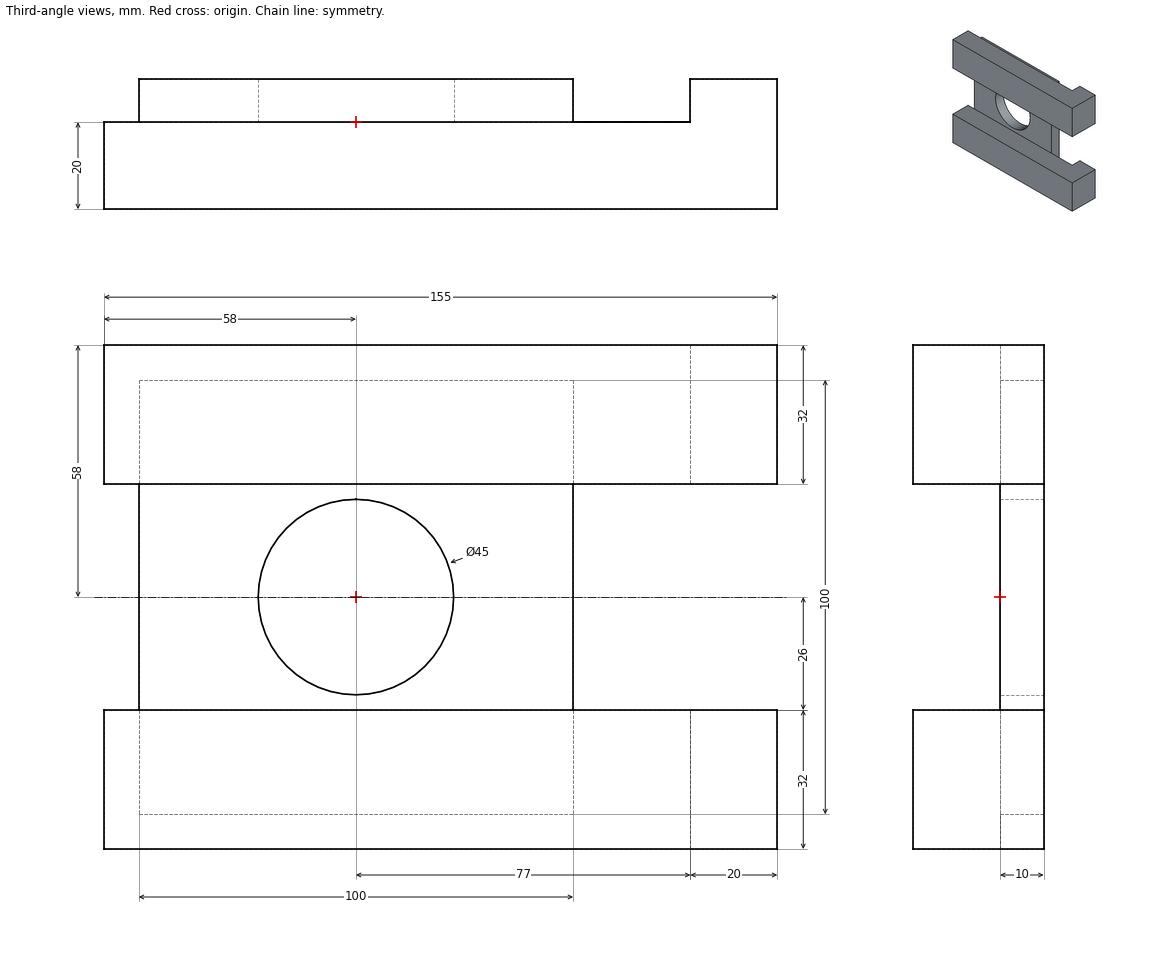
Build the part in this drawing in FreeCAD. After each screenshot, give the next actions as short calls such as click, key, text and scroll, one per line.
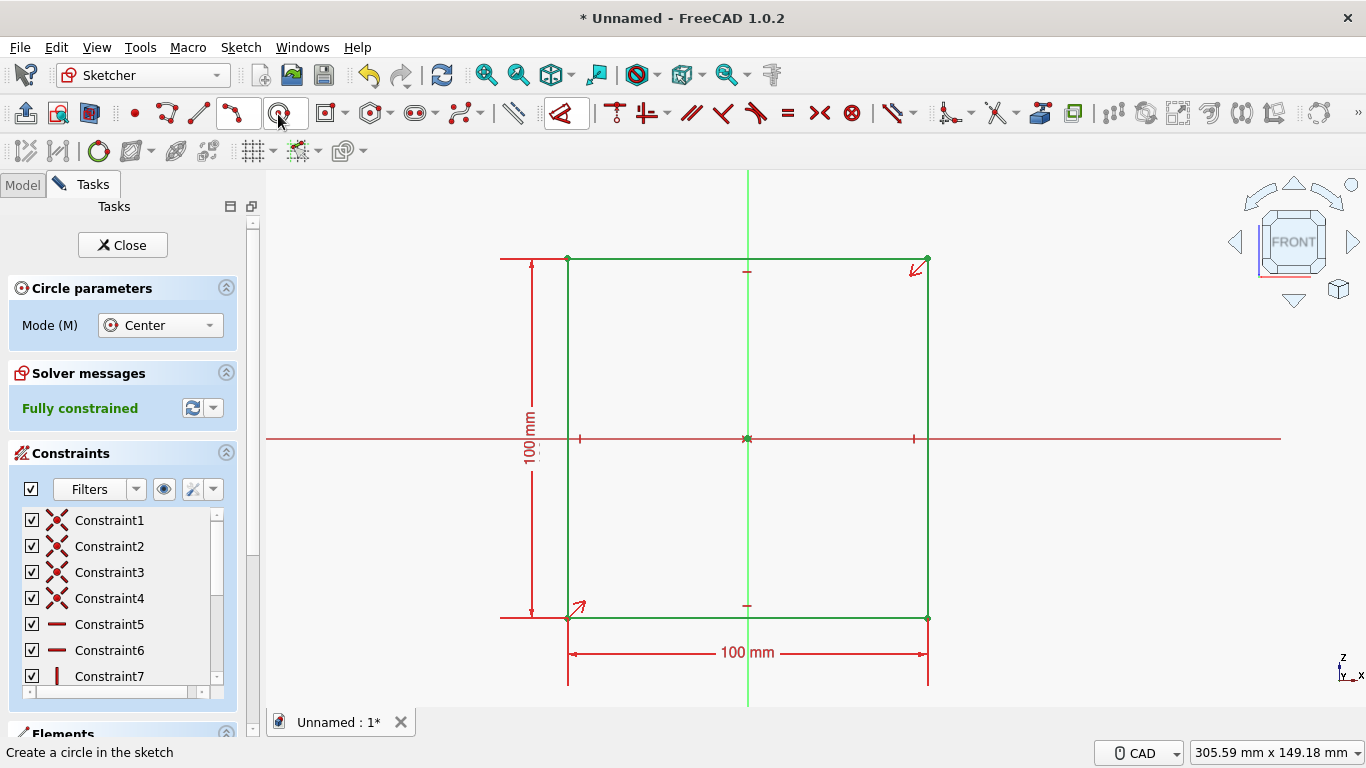
click(748, 438)
move(805, 381)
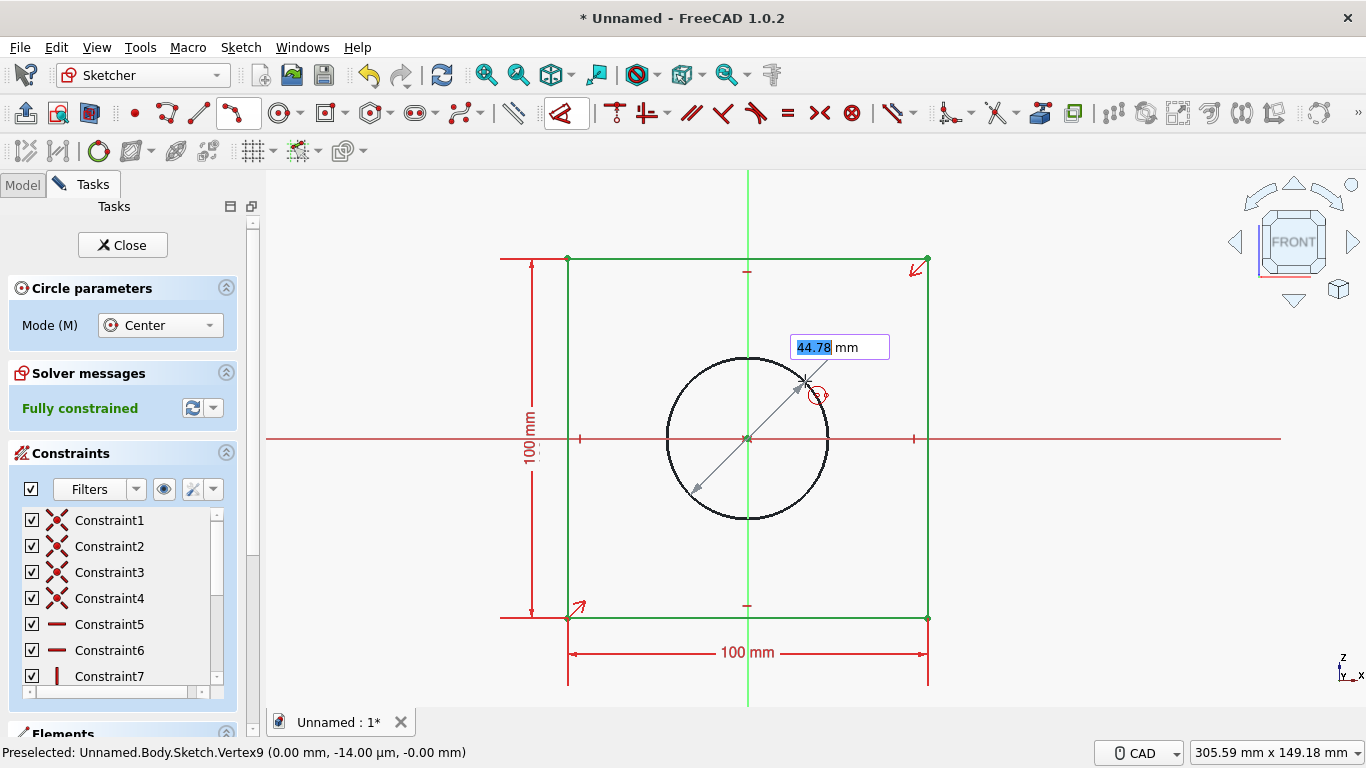
text(45)
key(Return)
key(Escape)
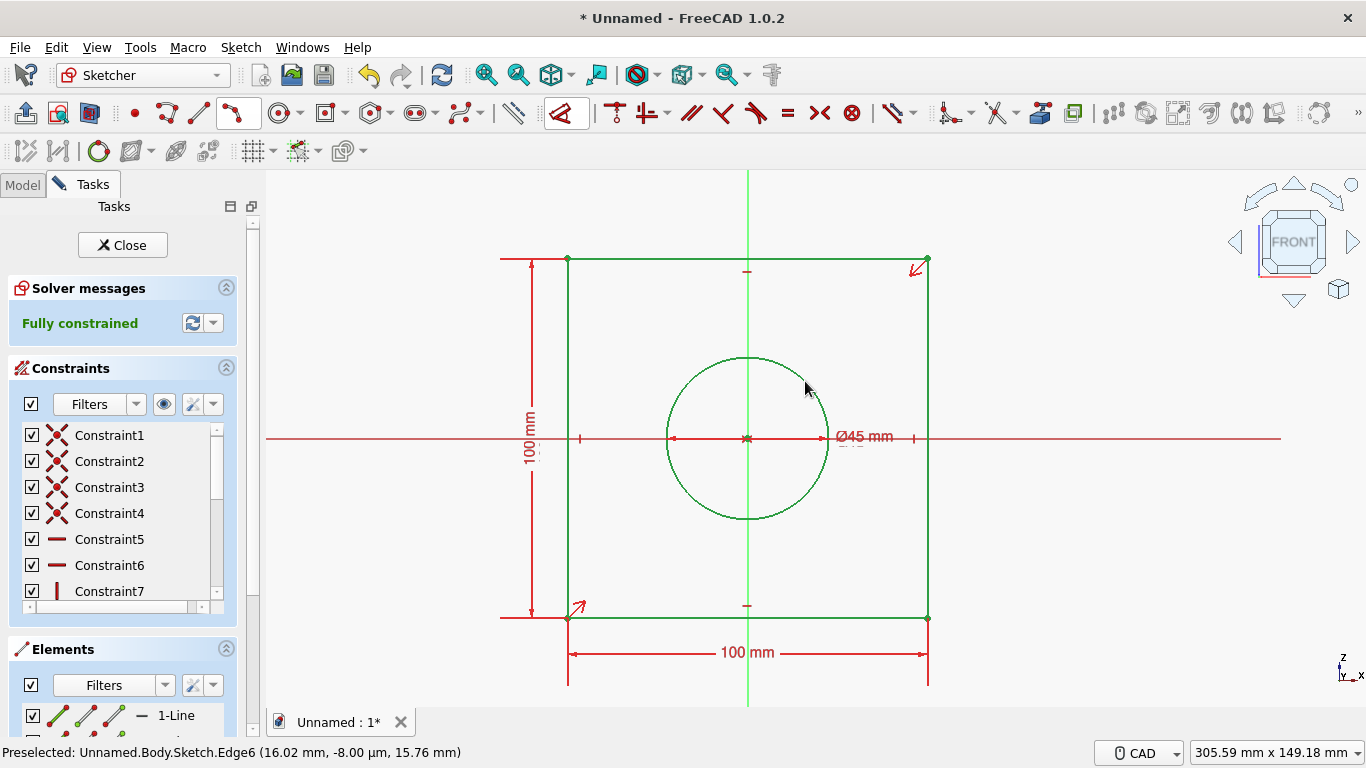
click(123, 245)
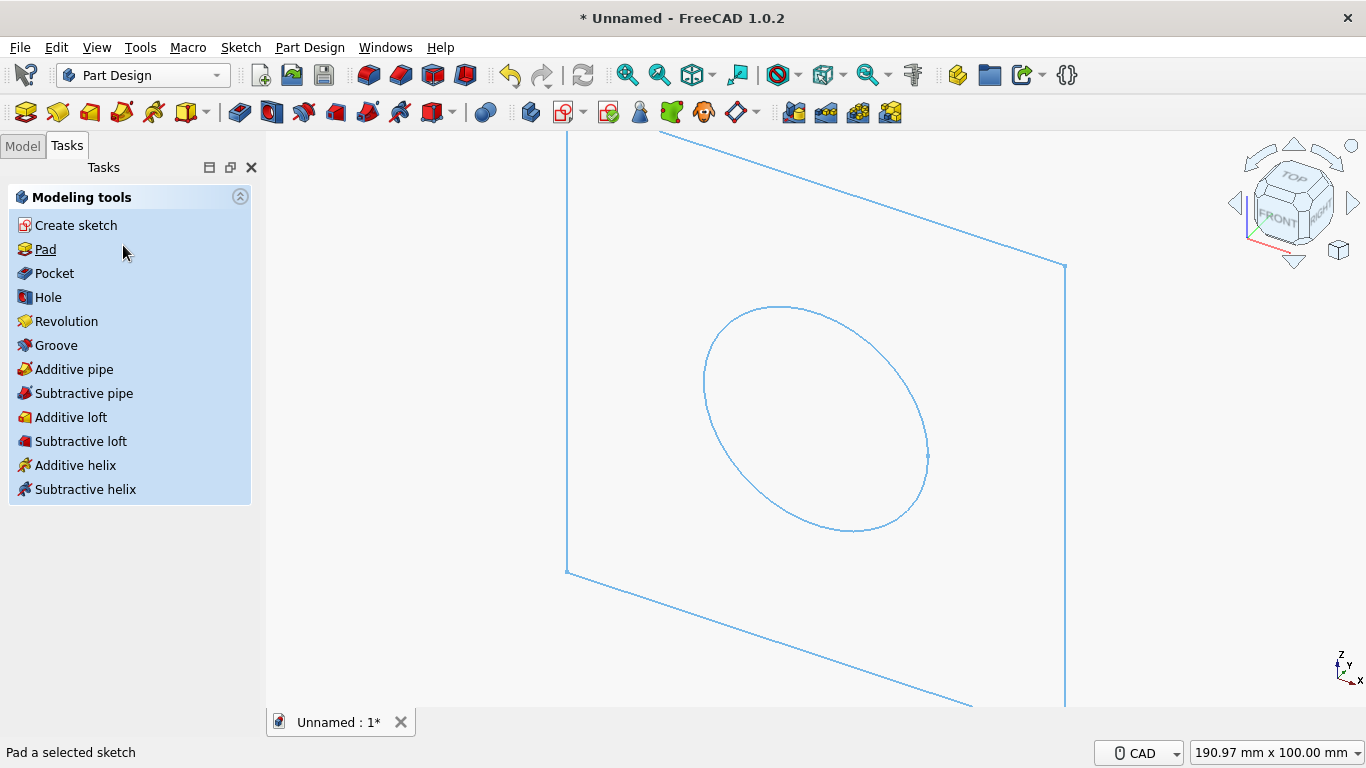
click(26, 112)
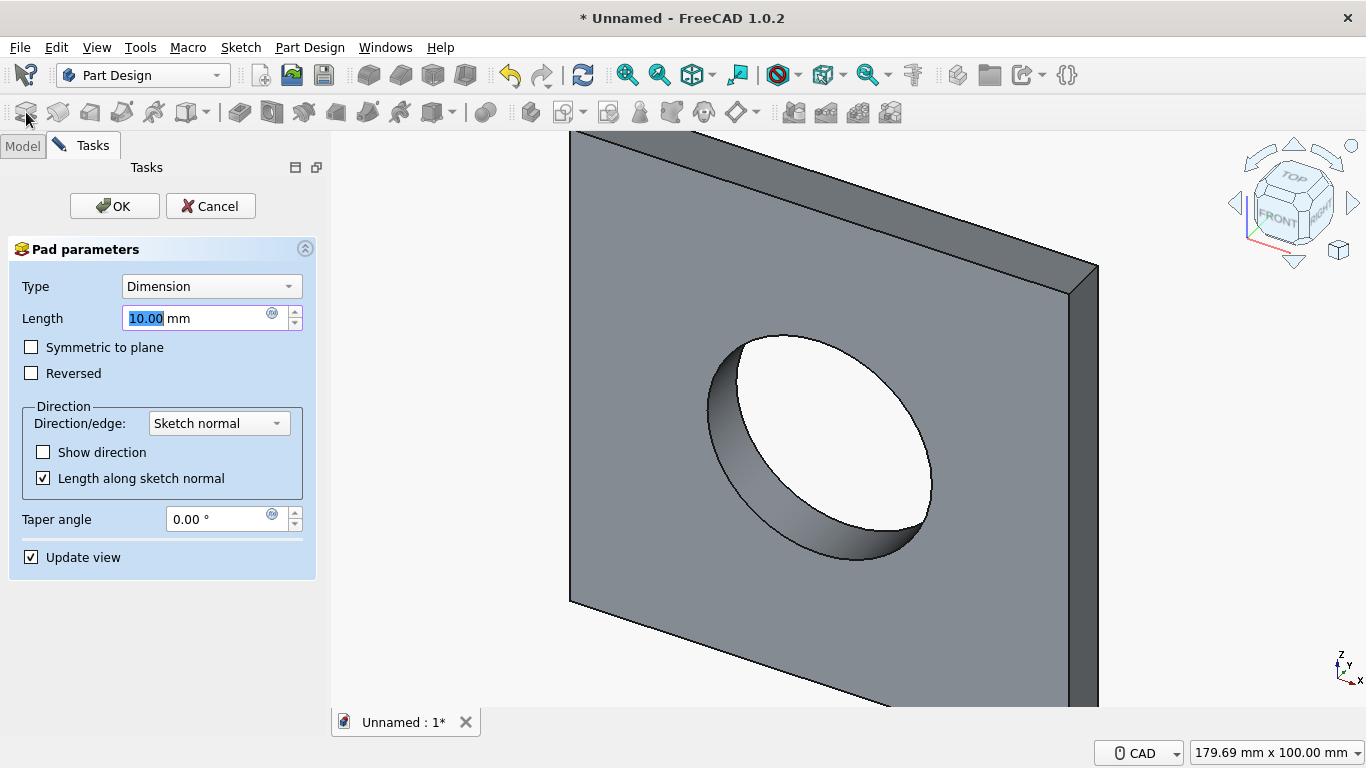
text(10)
key(Tab)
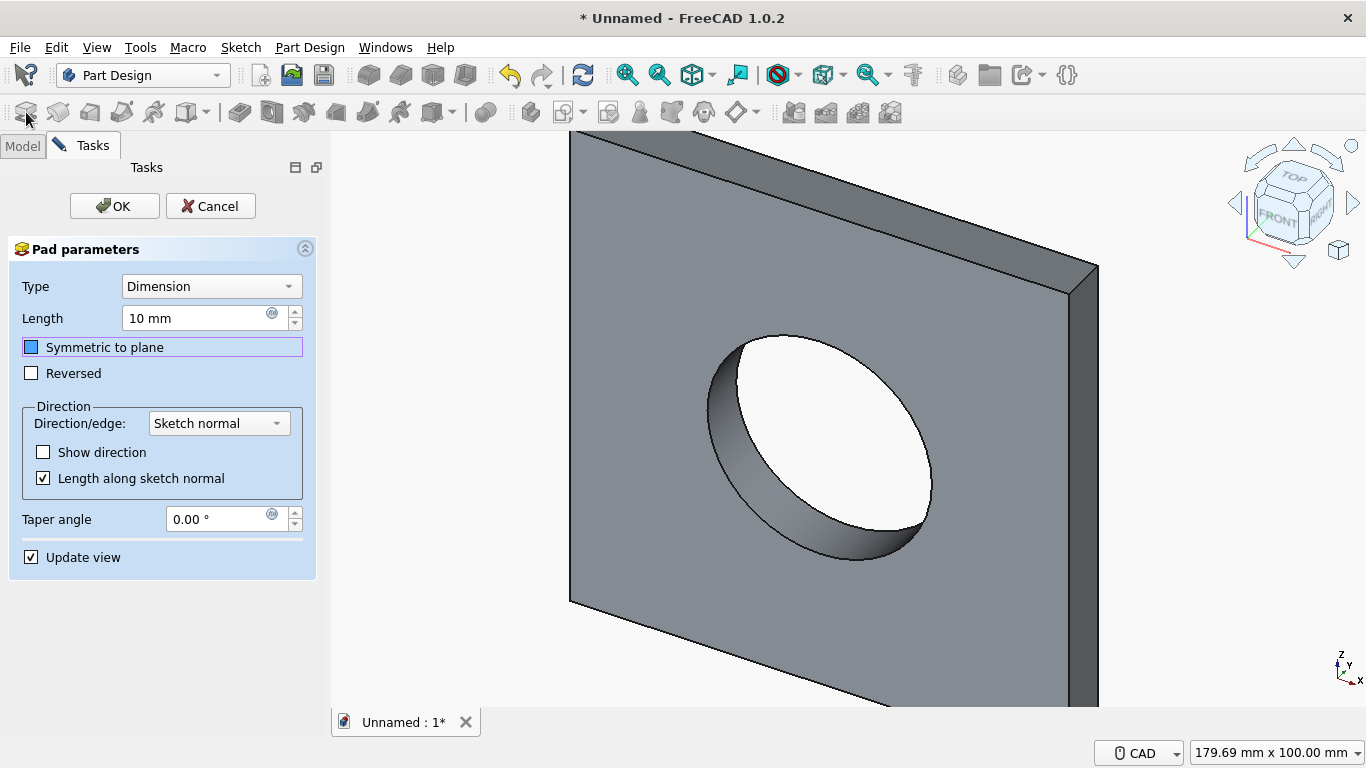
click(30, 373)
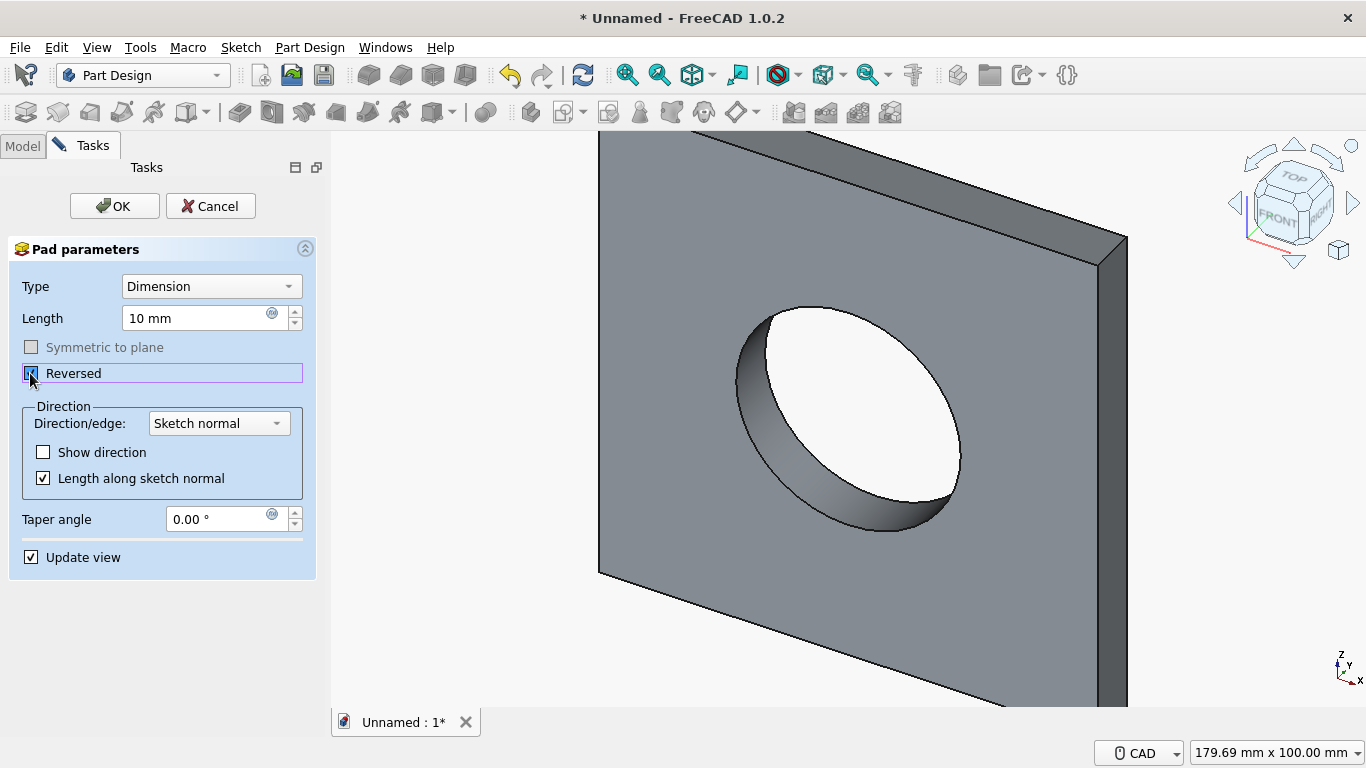
click(115, 206)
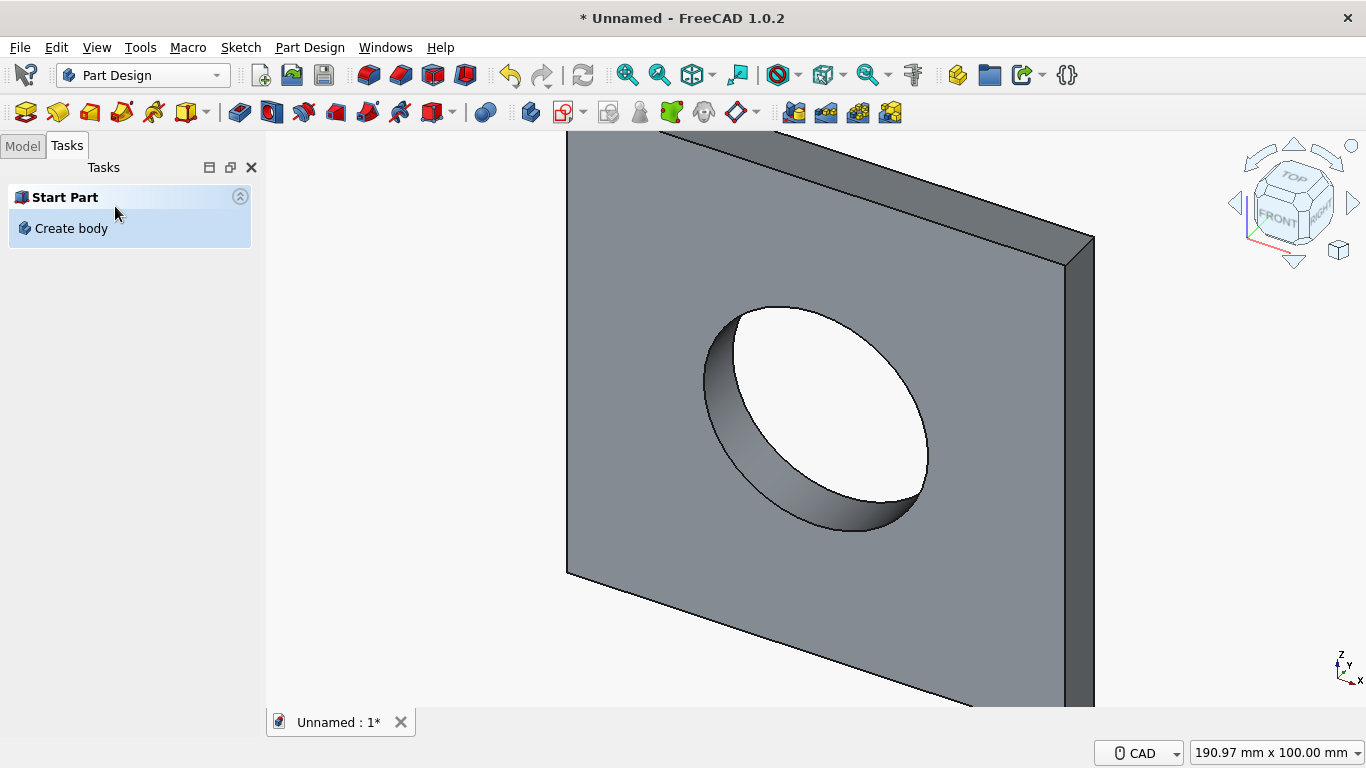
click(628, 76)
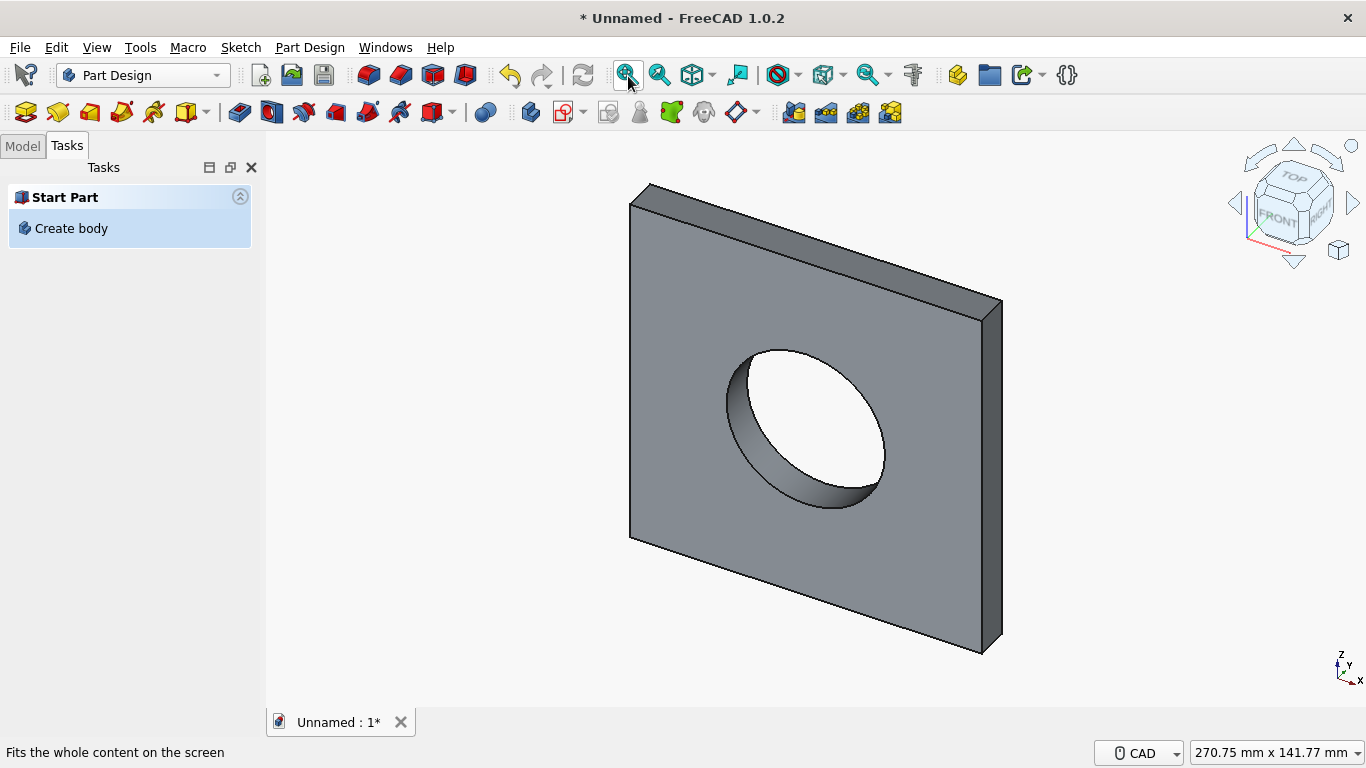
click(564, 112)